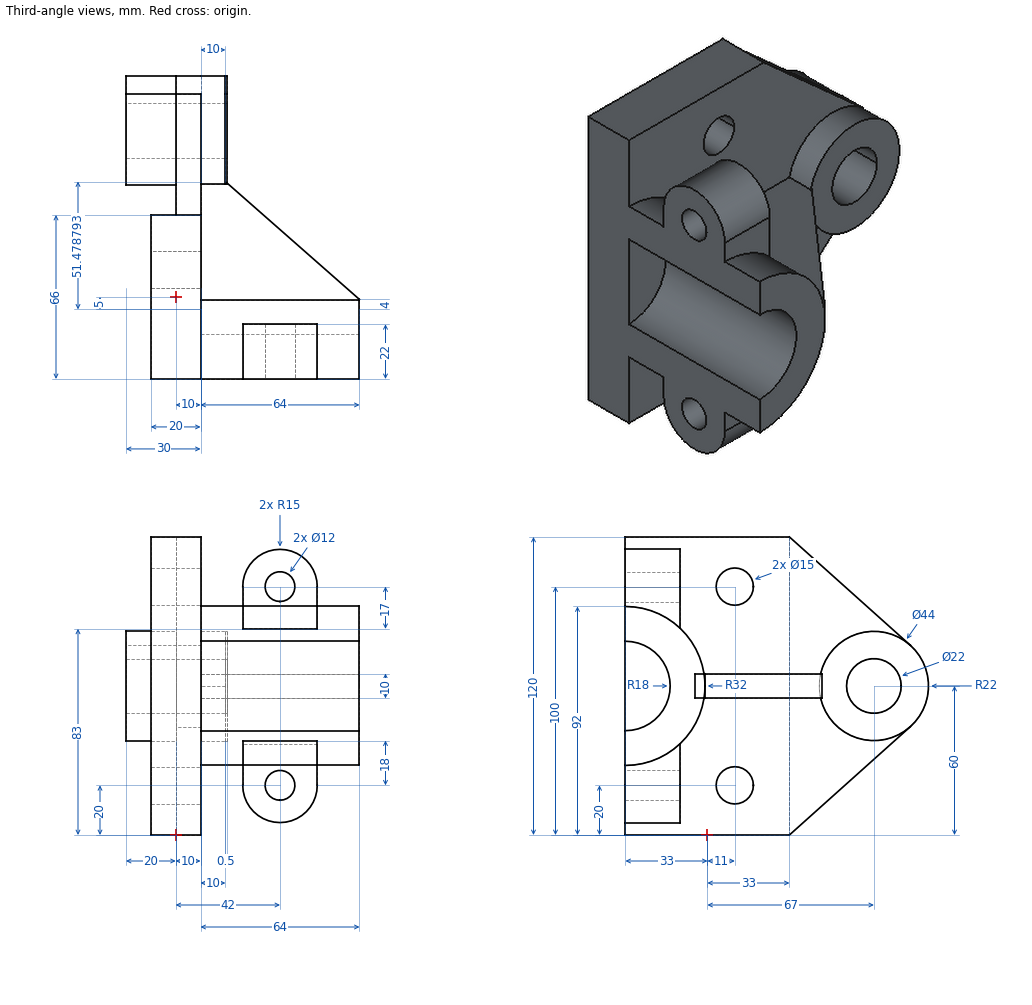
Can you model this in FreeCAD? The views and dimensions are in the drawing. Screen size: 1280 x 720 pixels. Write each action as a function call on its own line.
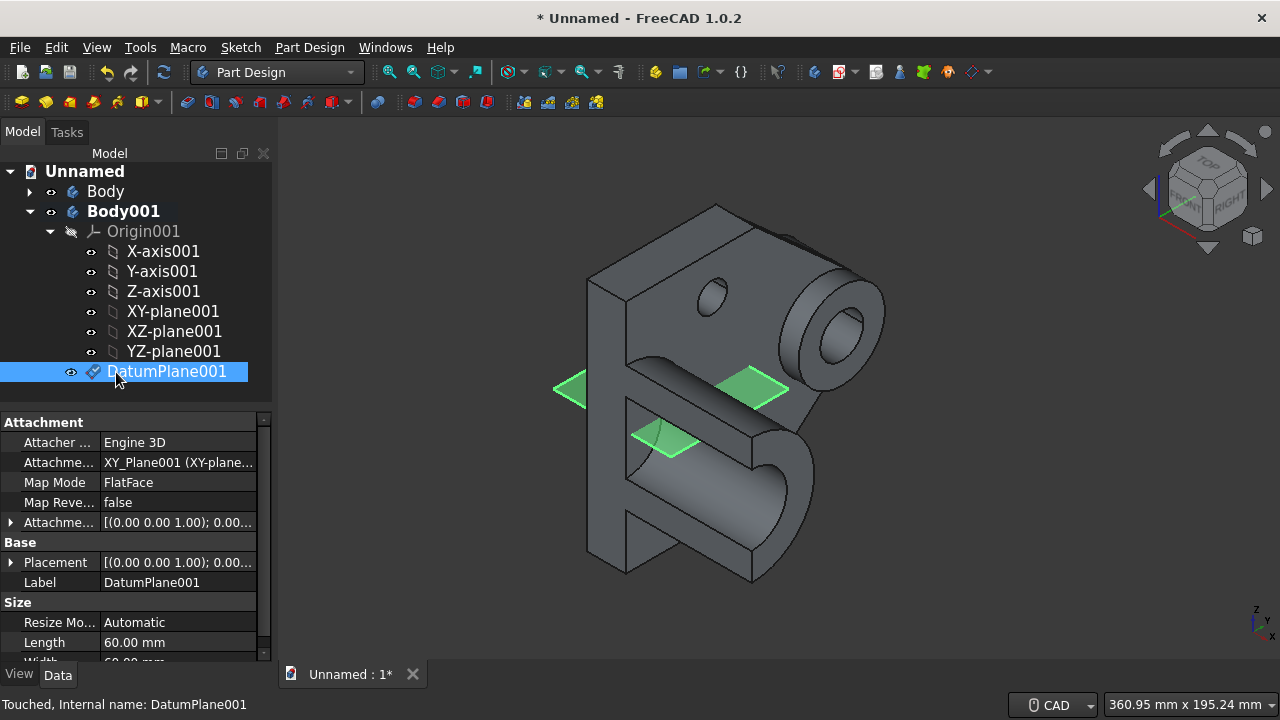
click(840, 72)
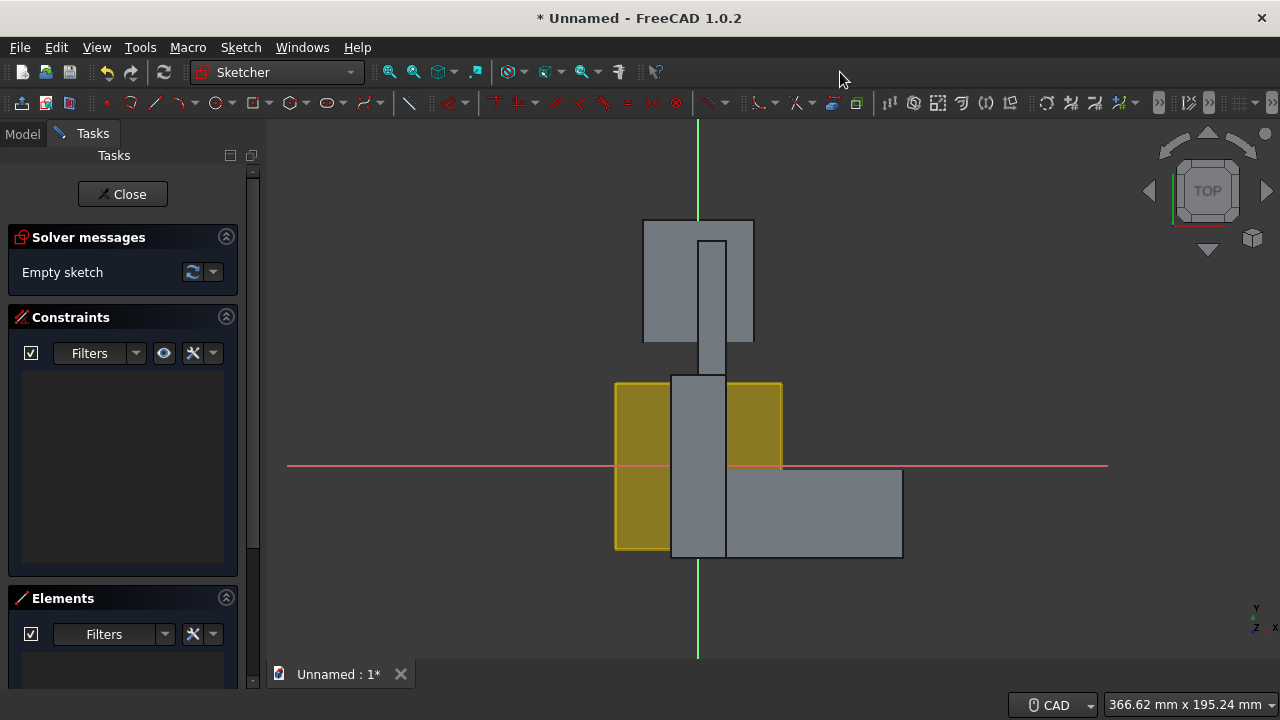
scroll(879, 425, up, 4)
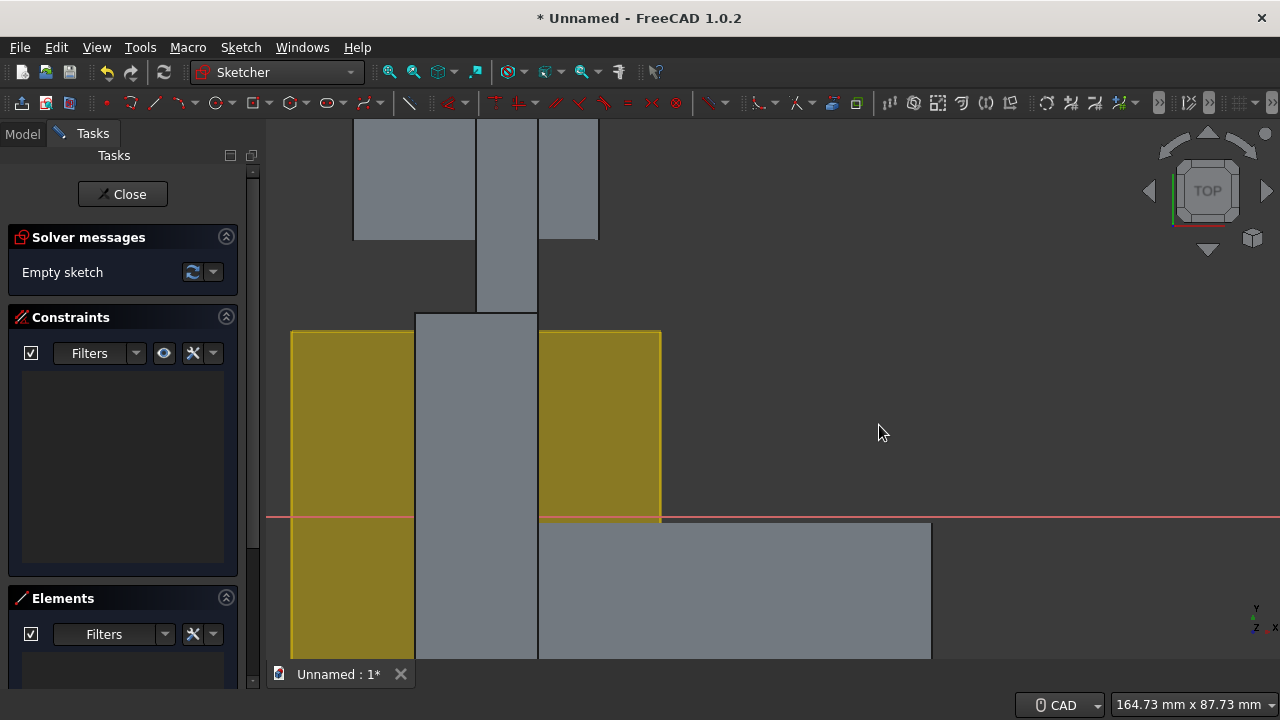
click(132, 104)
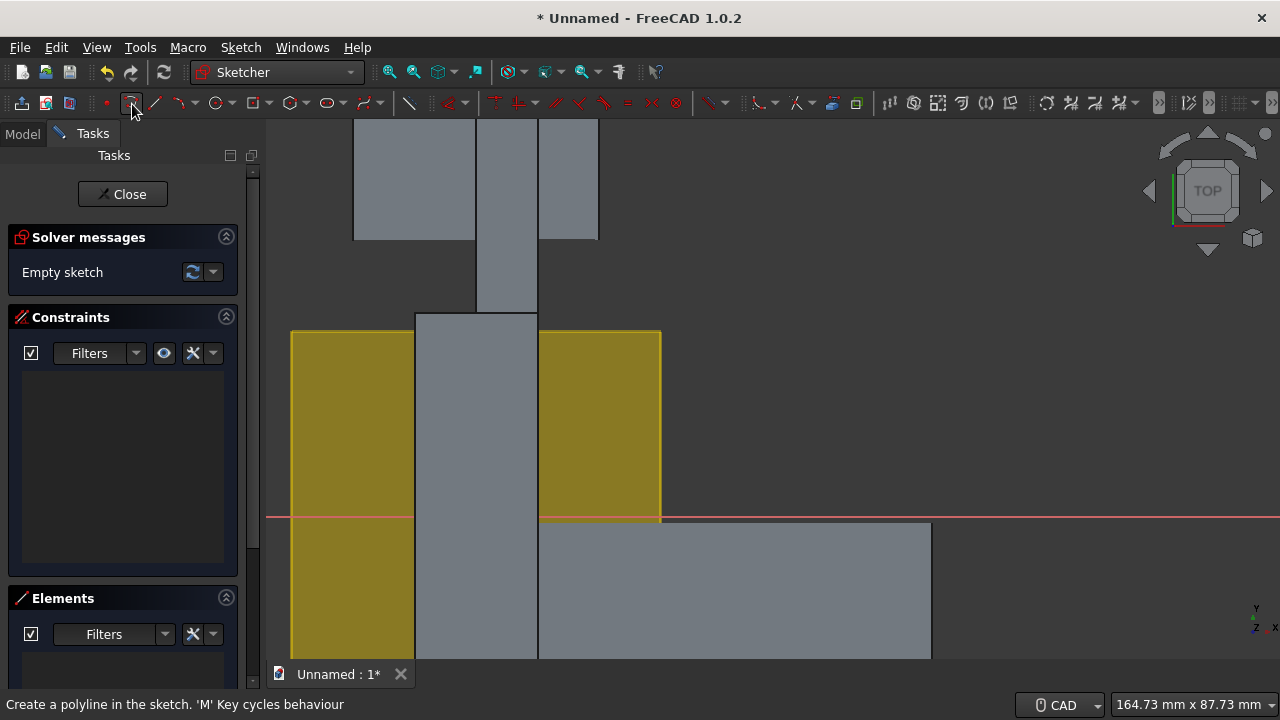
click(538, 547)
click(932, 547)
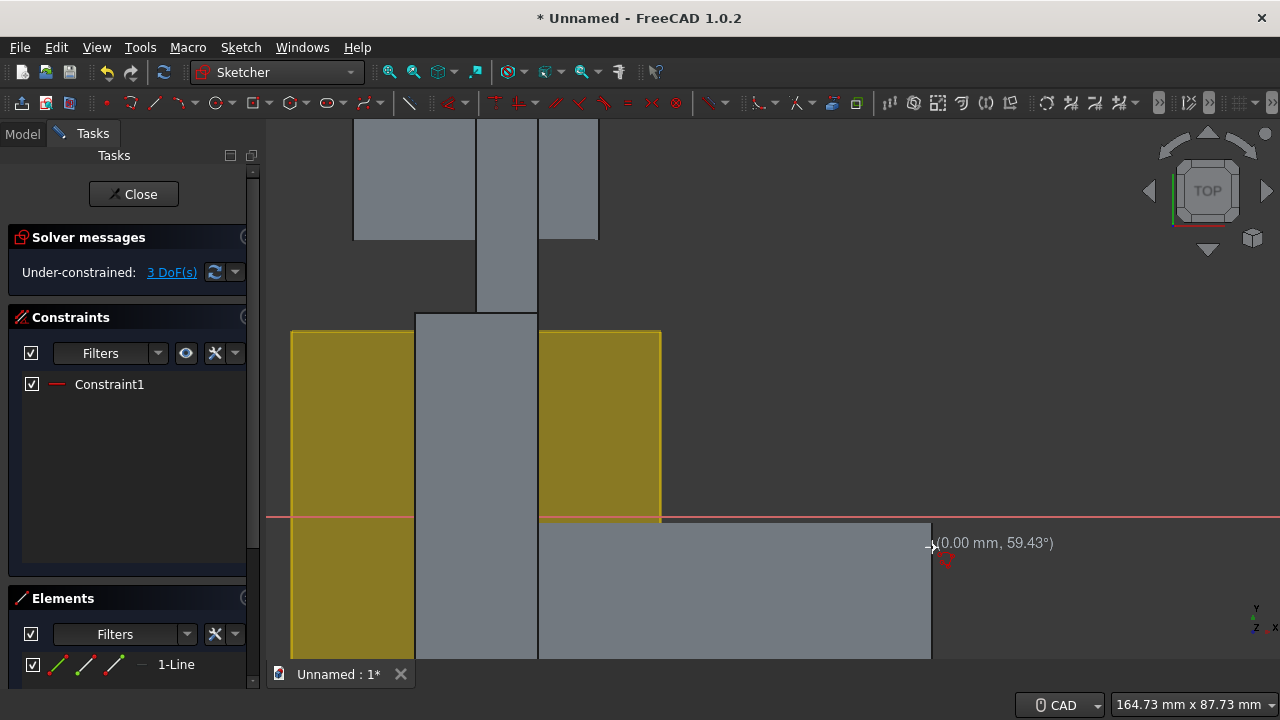
scroll(932, 523, up, 5)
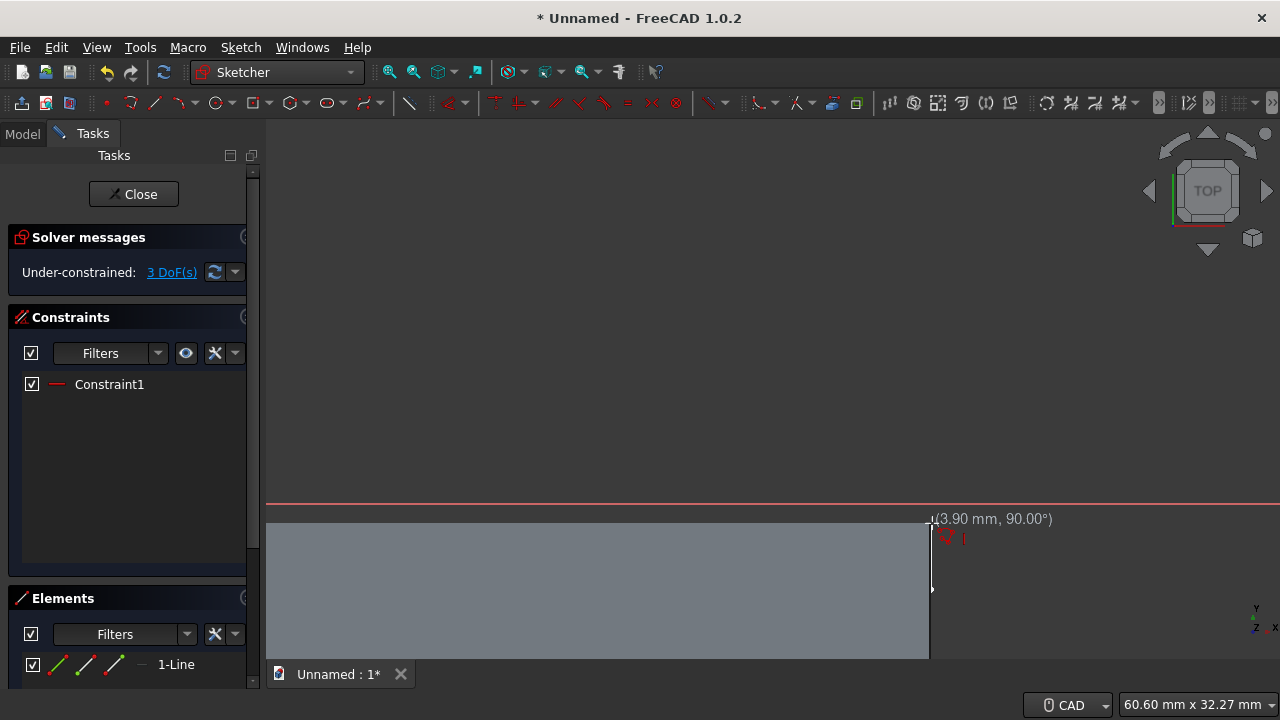
click(931, 521)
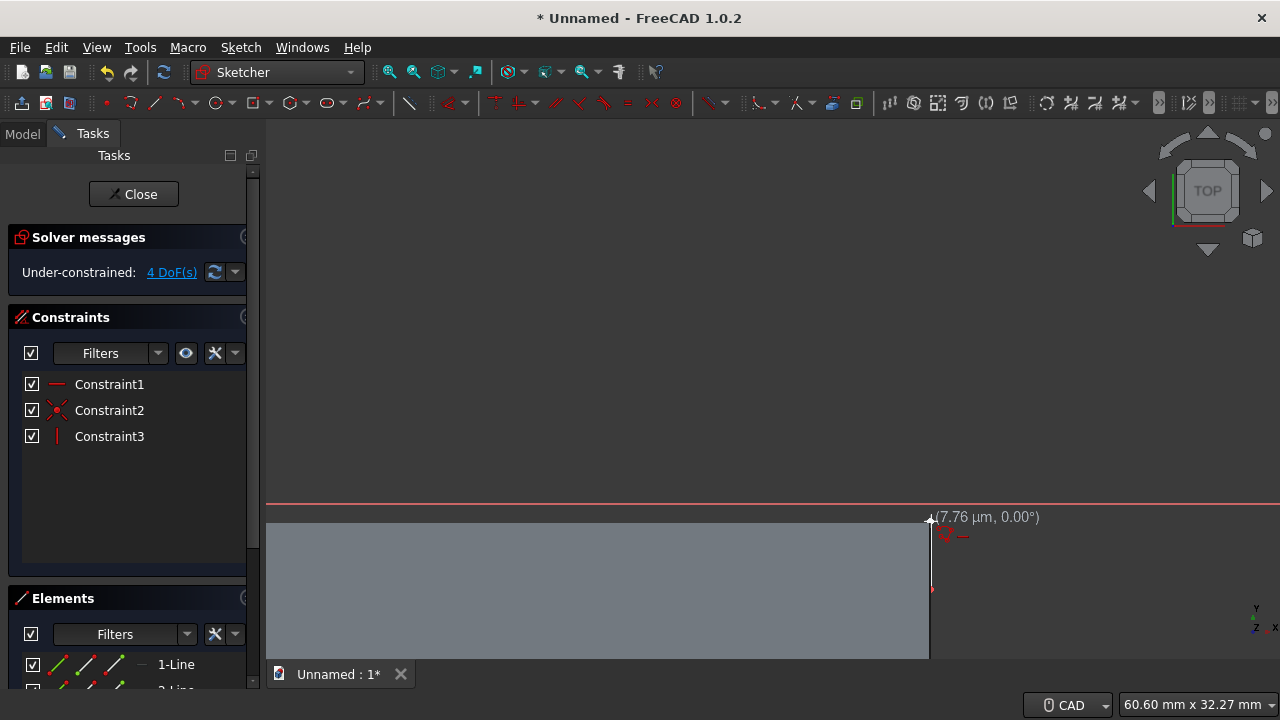
scroll(934, 524, down, 5)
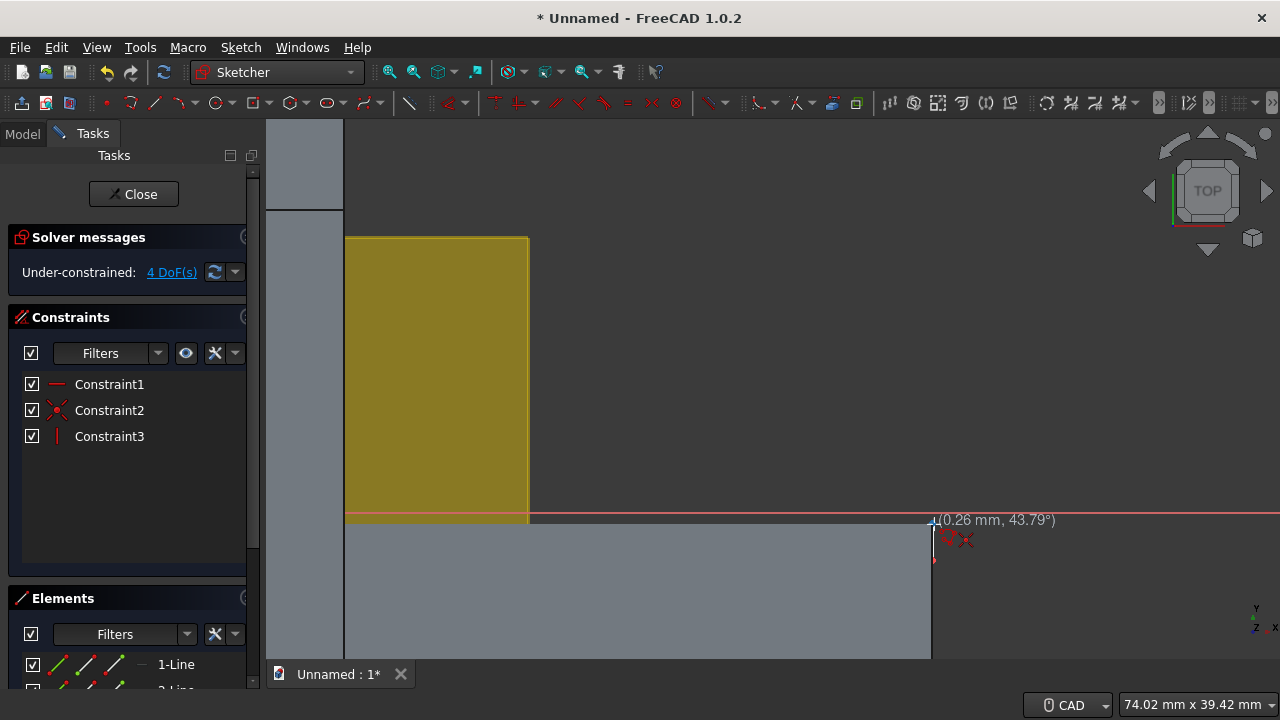
click(601, 231)
click(539, 231)
click(539, 549)
key(Escape)
key(Escape)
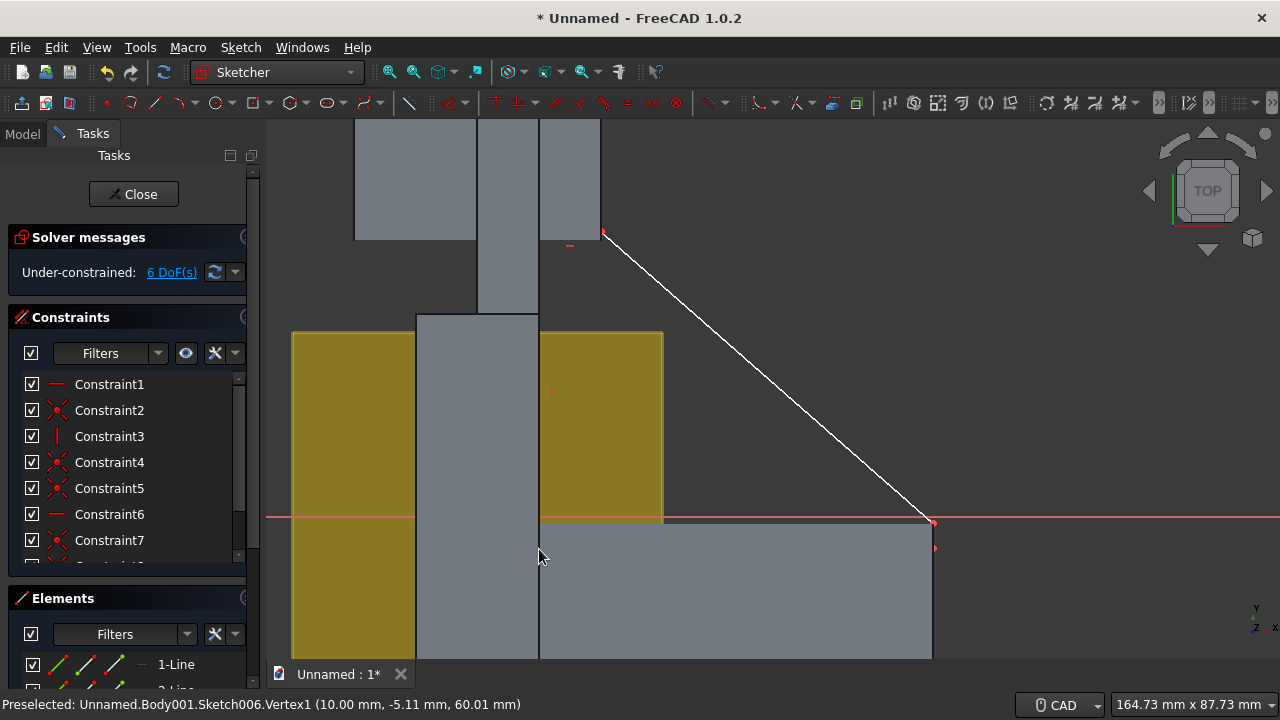
click(448, 104)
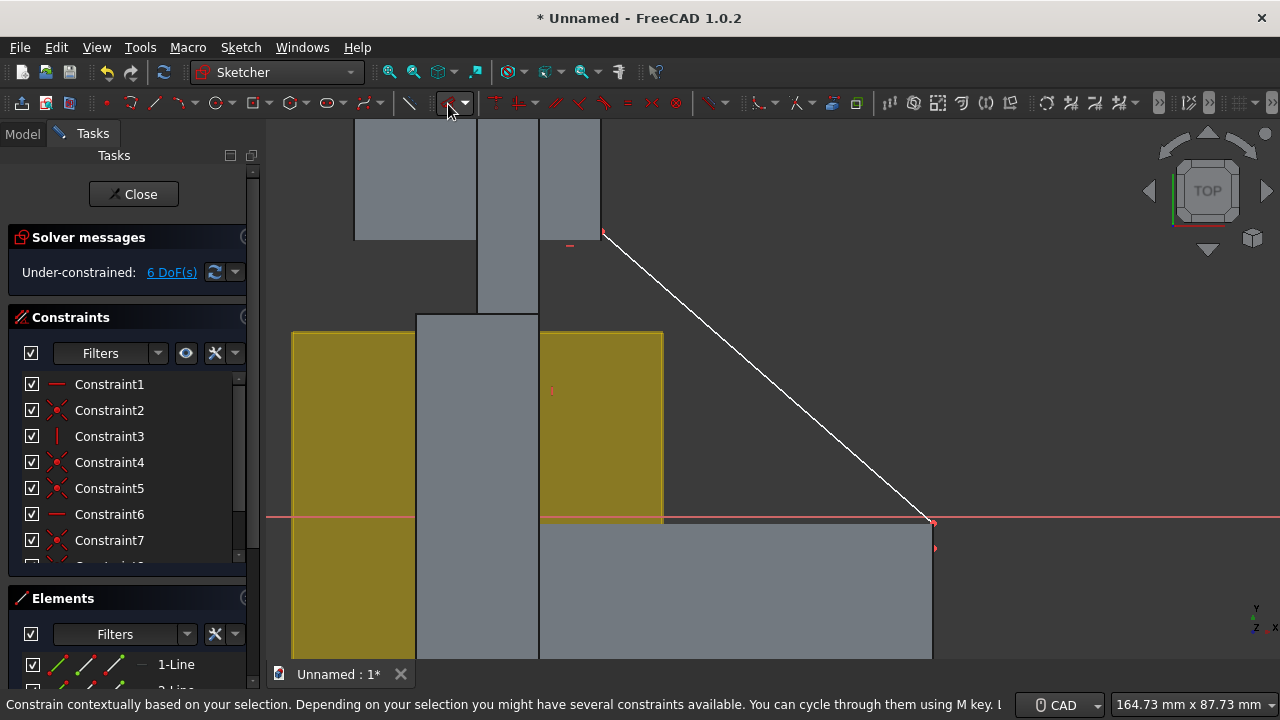
scroll(933, 539, up, 3)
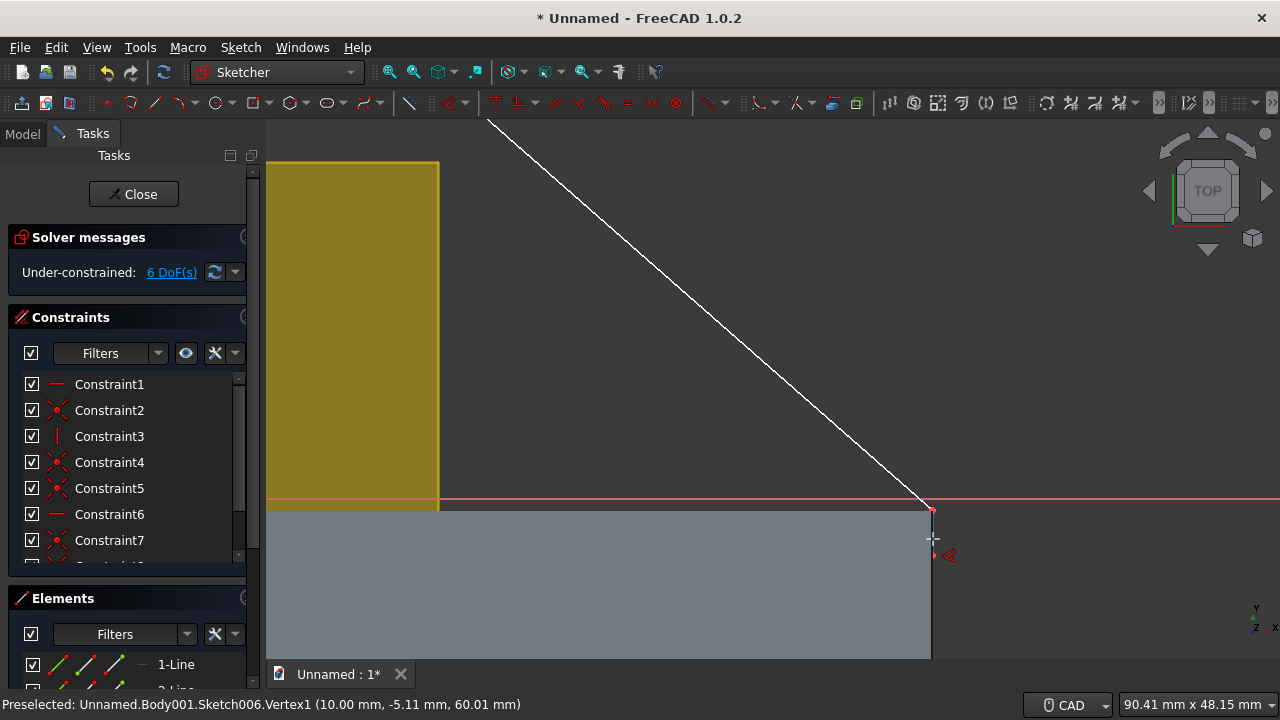
click(933, 538)
click(967, 533)